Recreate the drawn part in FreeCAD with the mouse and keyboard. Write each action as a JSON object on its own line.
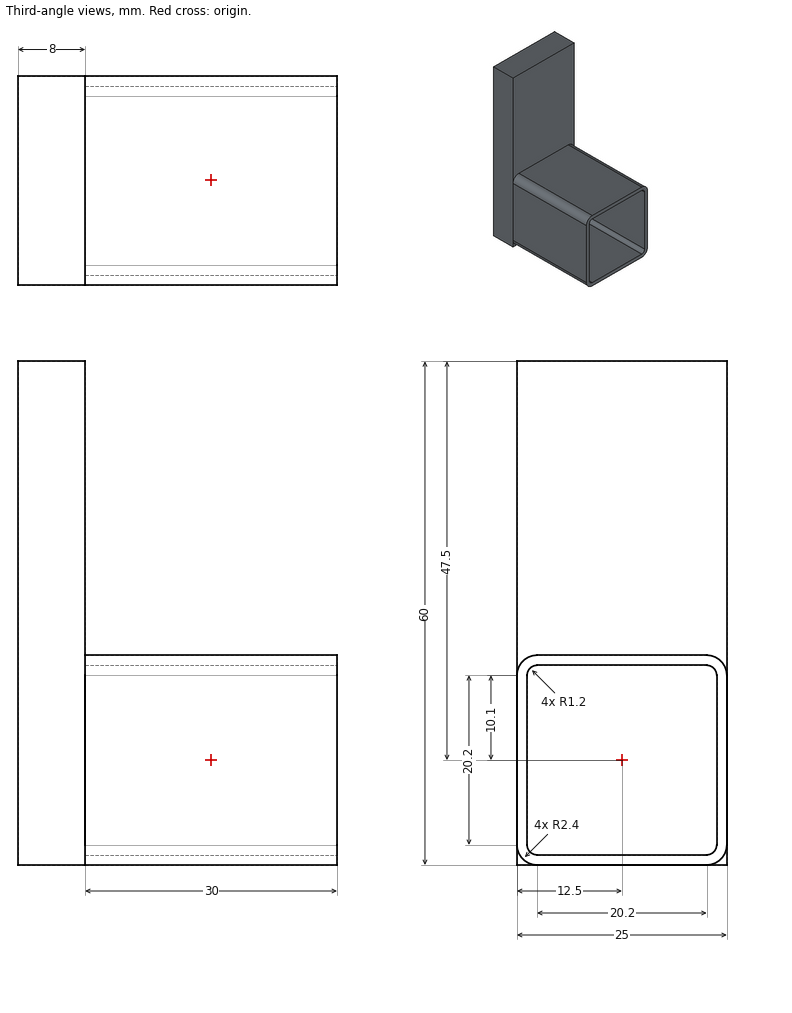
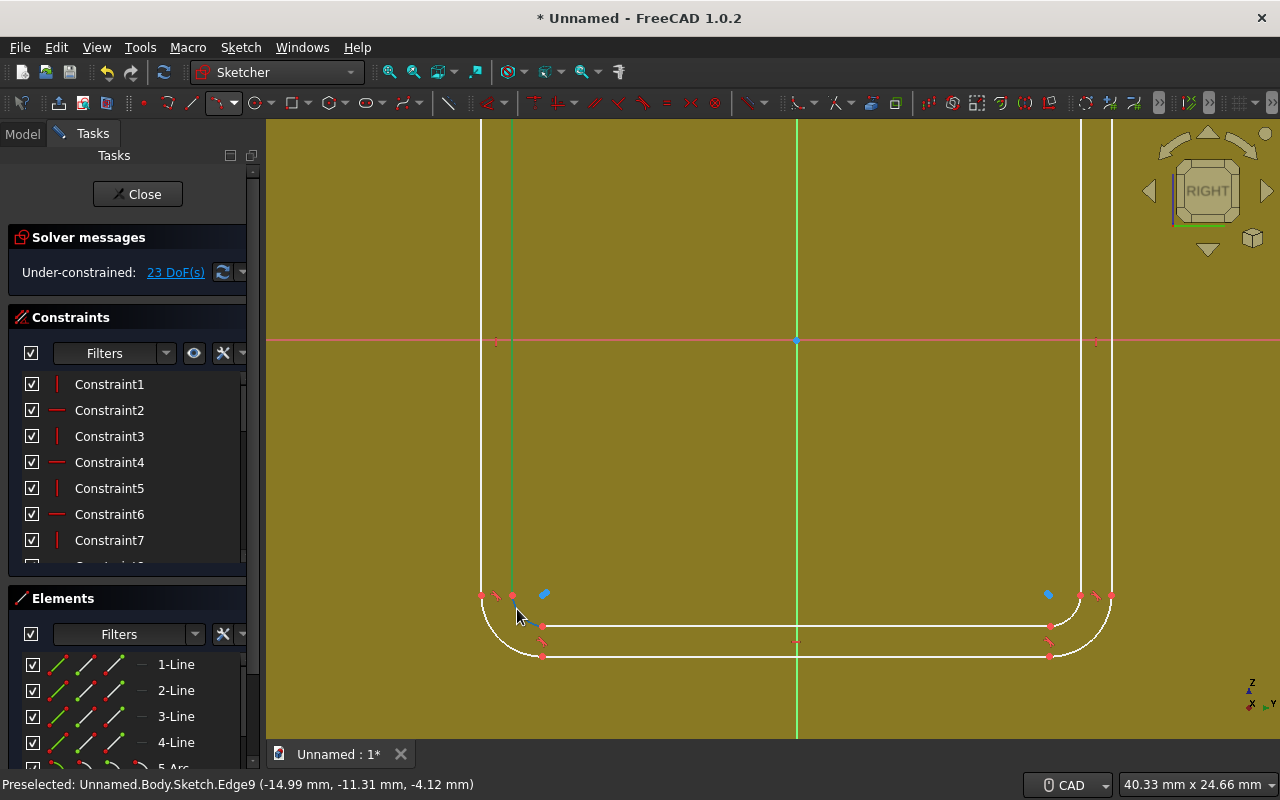
{"action": "left_click", "coordinate": [516, 609]}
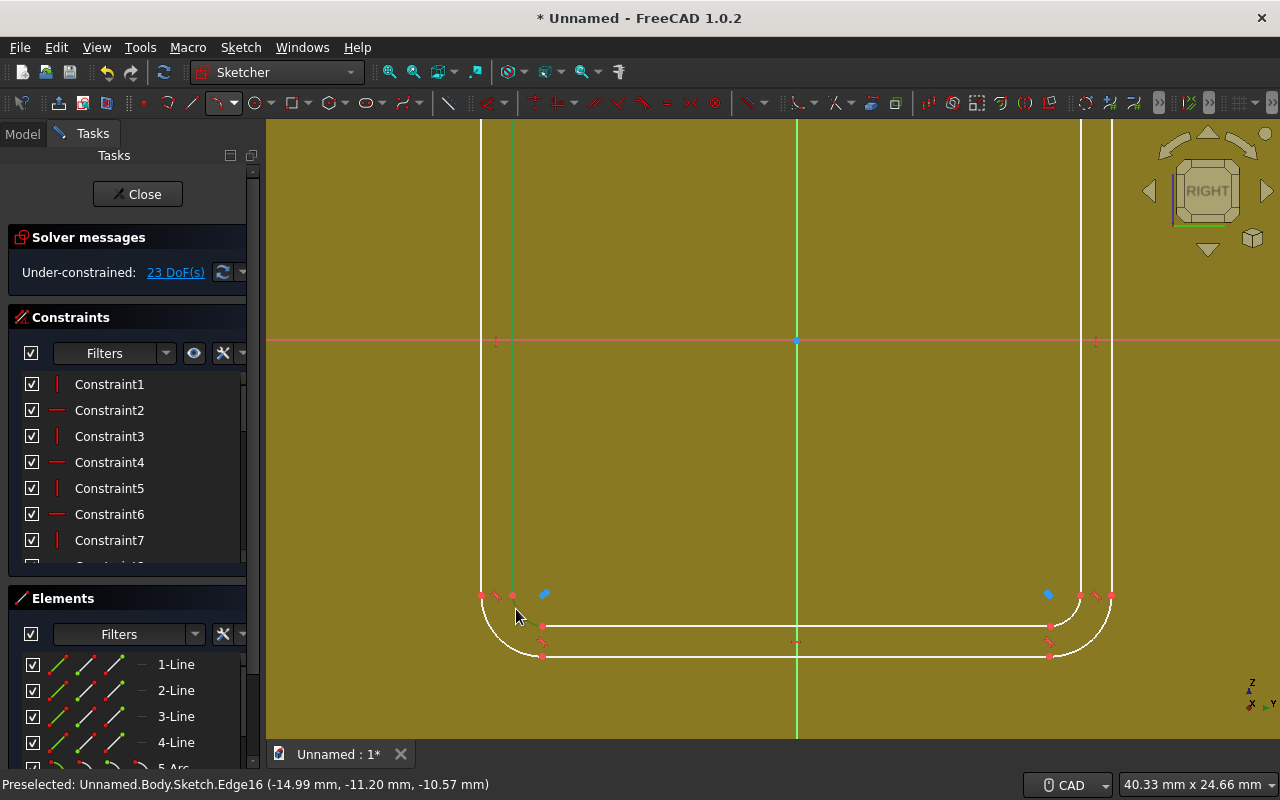
{"action": "key", "text": "t"}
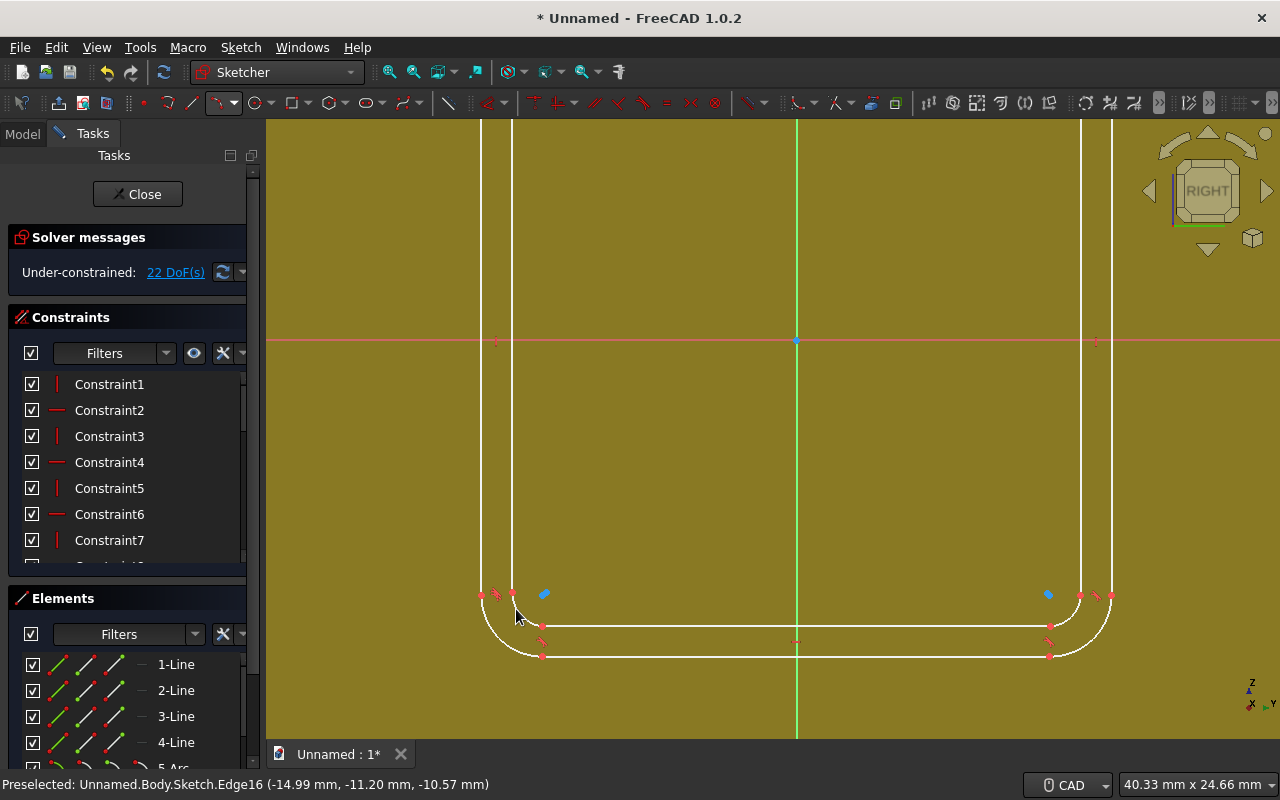
{"action": "scroll", "coordinate": [517, 609], "scroll_direction": "down", "scroll_amount": 2}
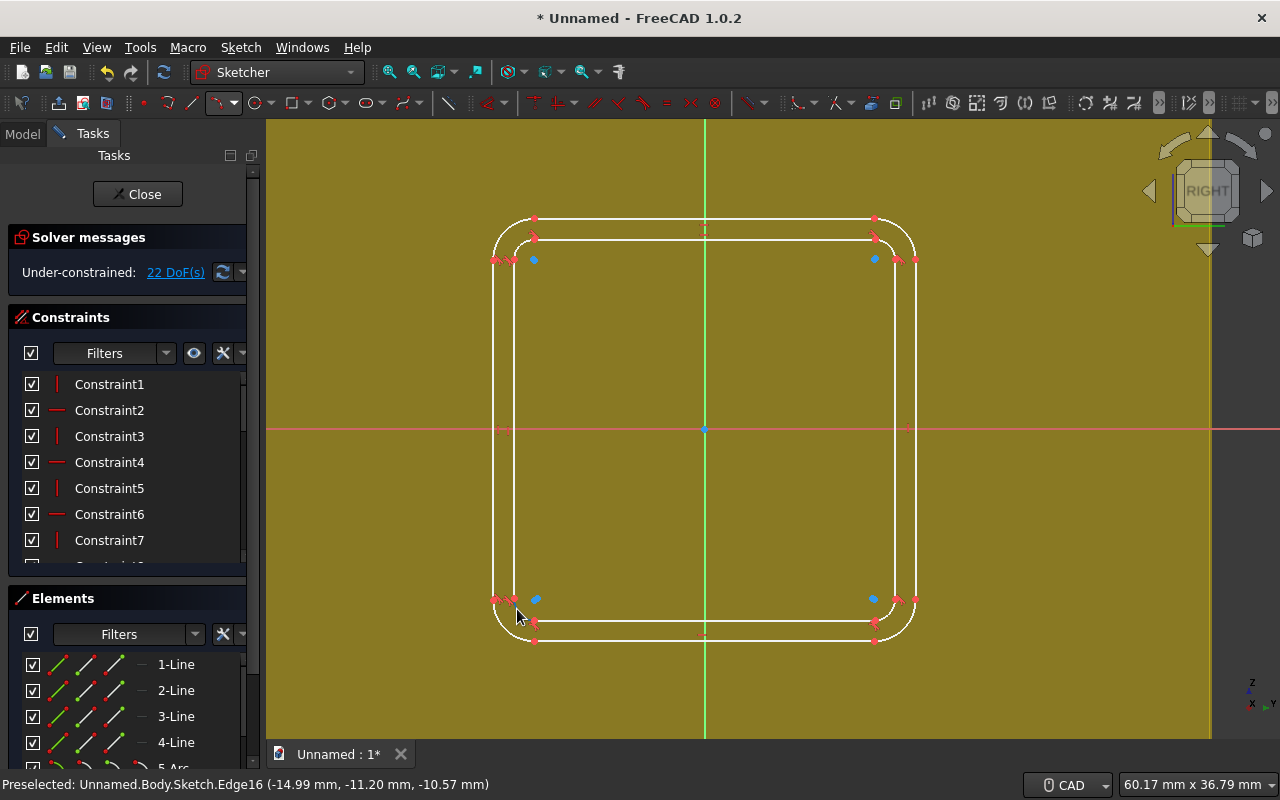
{"action": "left_click", "coordinate": [636, 240]}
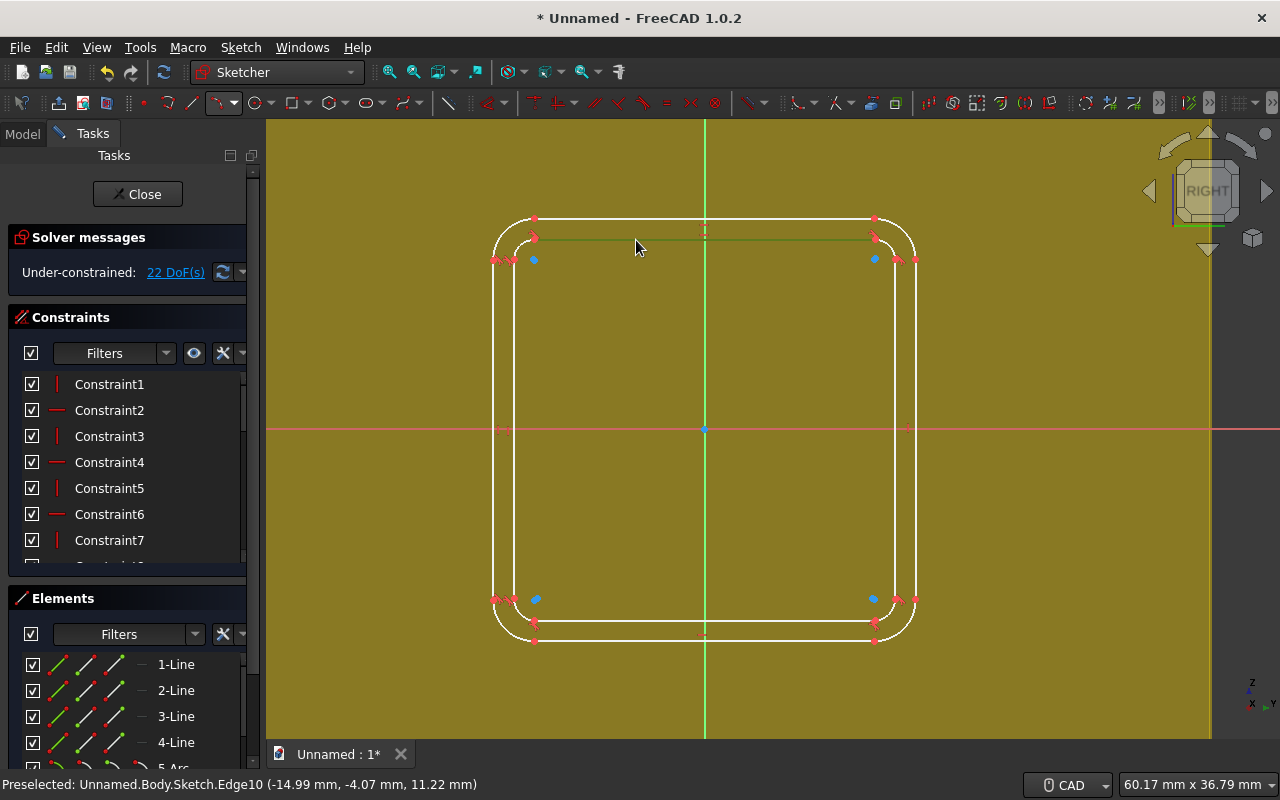
{"action": "scroll", "coordinate": [525, 242], "scroll_direction": "up", "scroll_amount": 2}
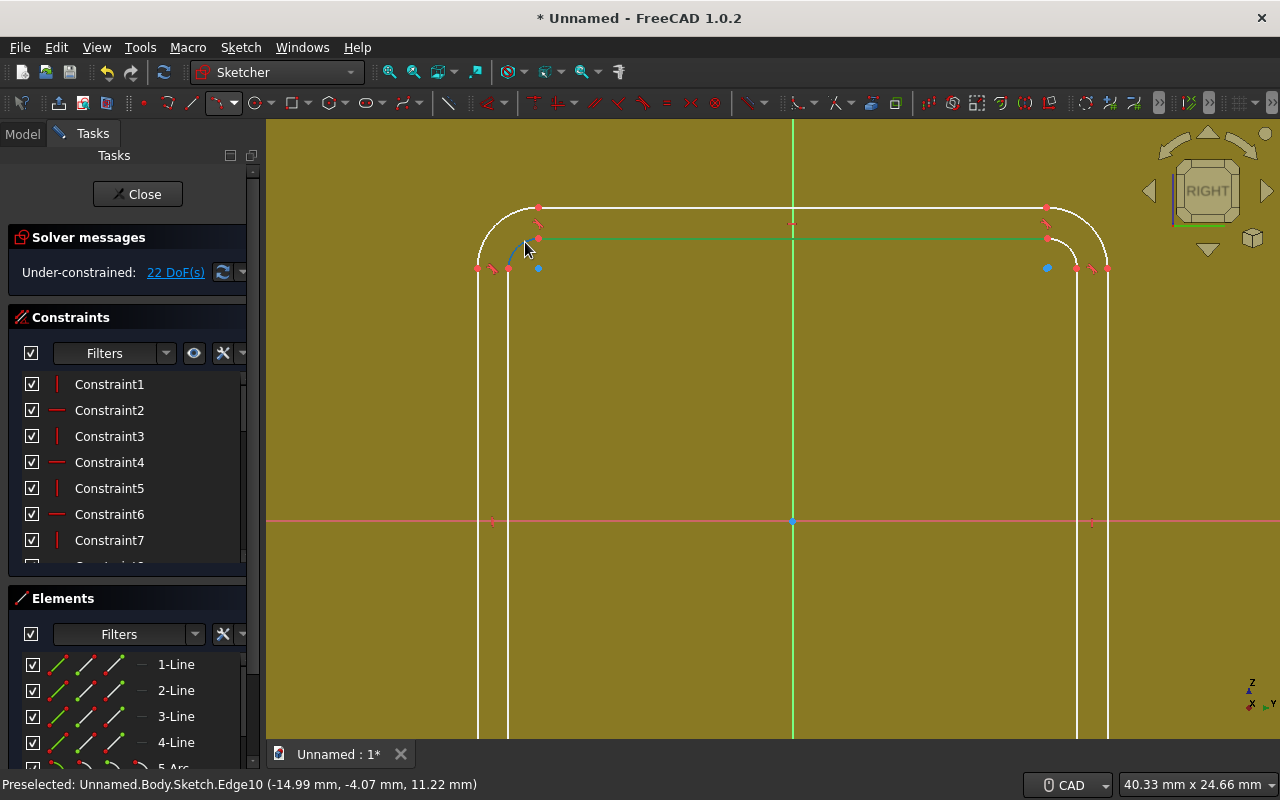
{"action": "left_click", "coordinate": [525, 242]}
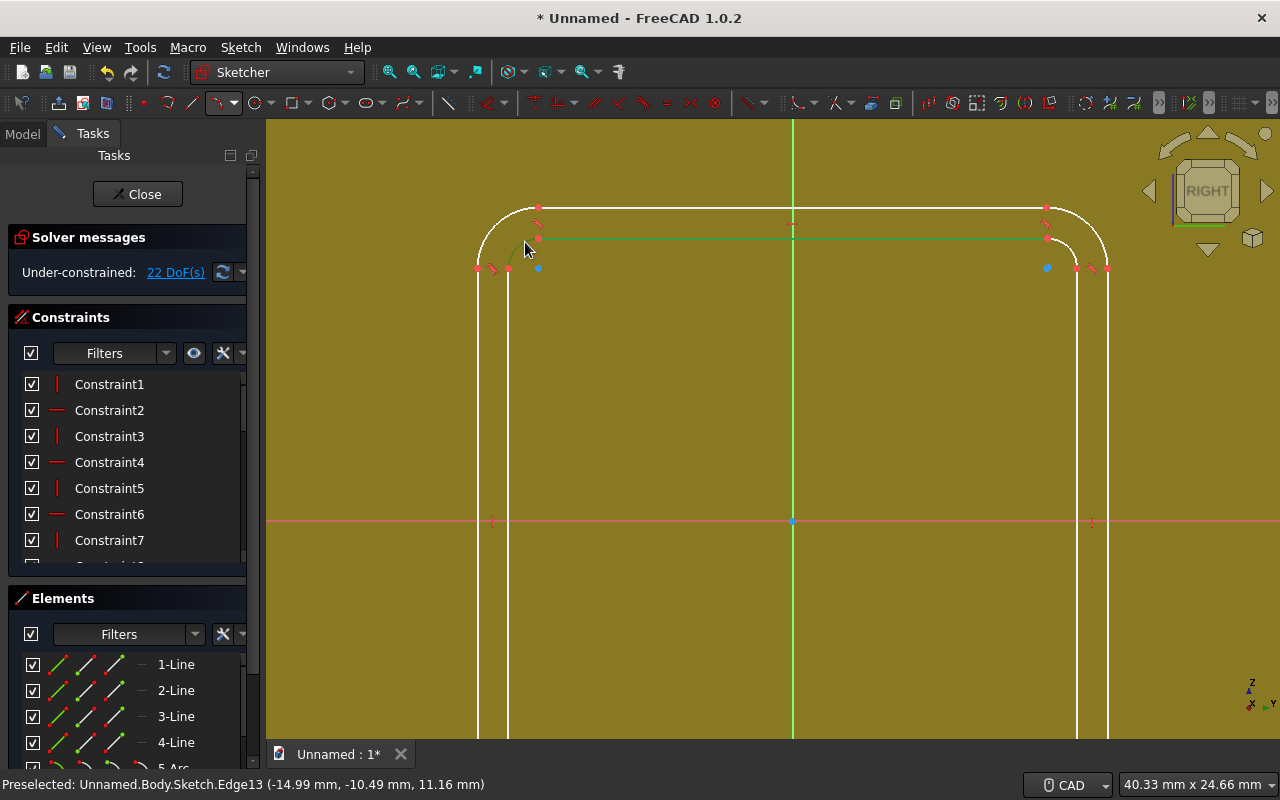
{"action": "left_click", "coordinate": [644, 104]}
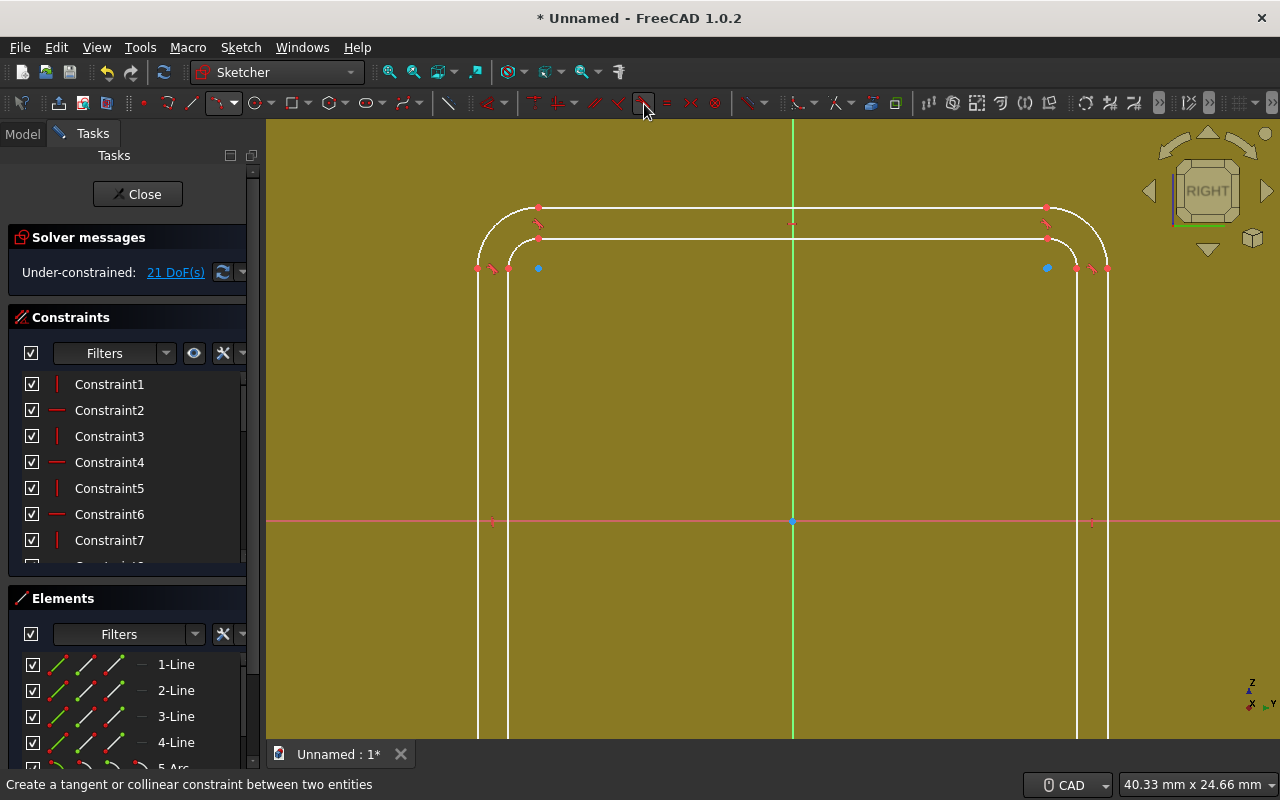
{"action": "left_click", "coordinate": [691, 239]}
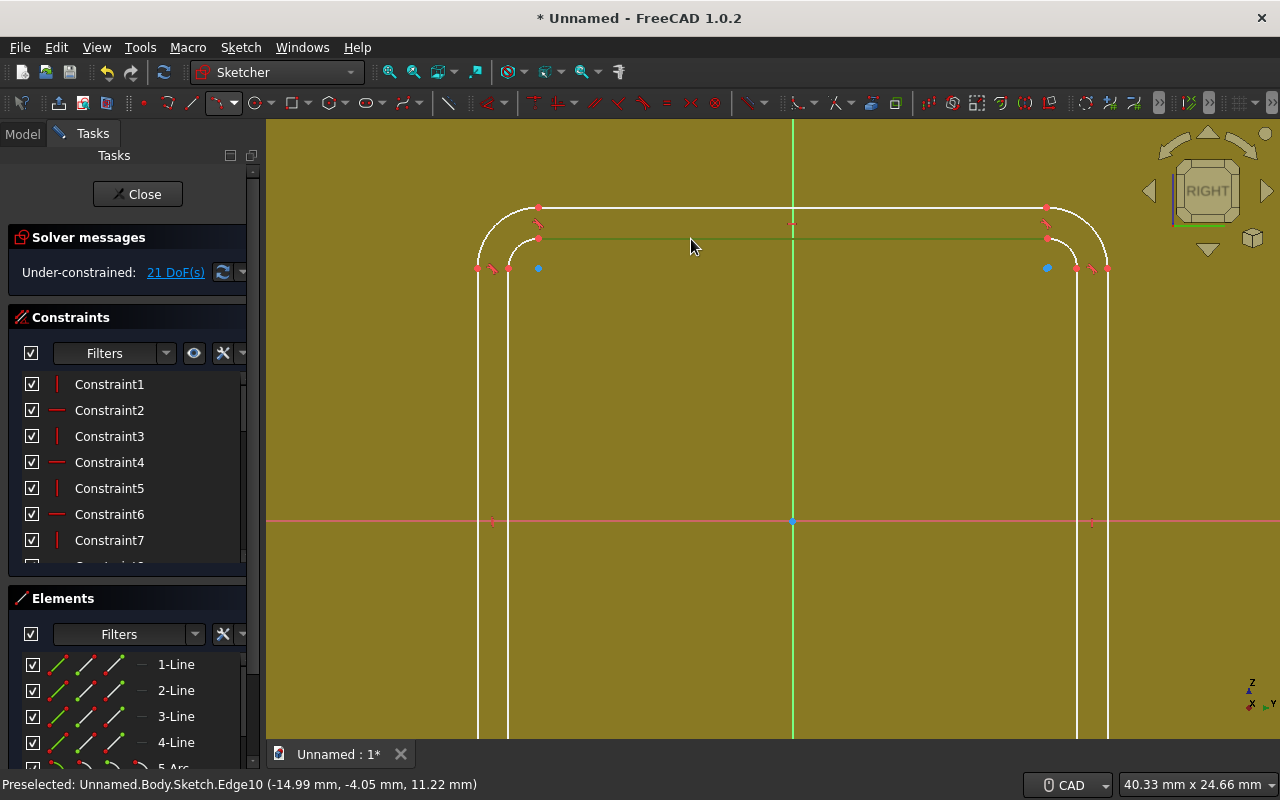
{"action": "left_click", "coordinate": [1074, 255]}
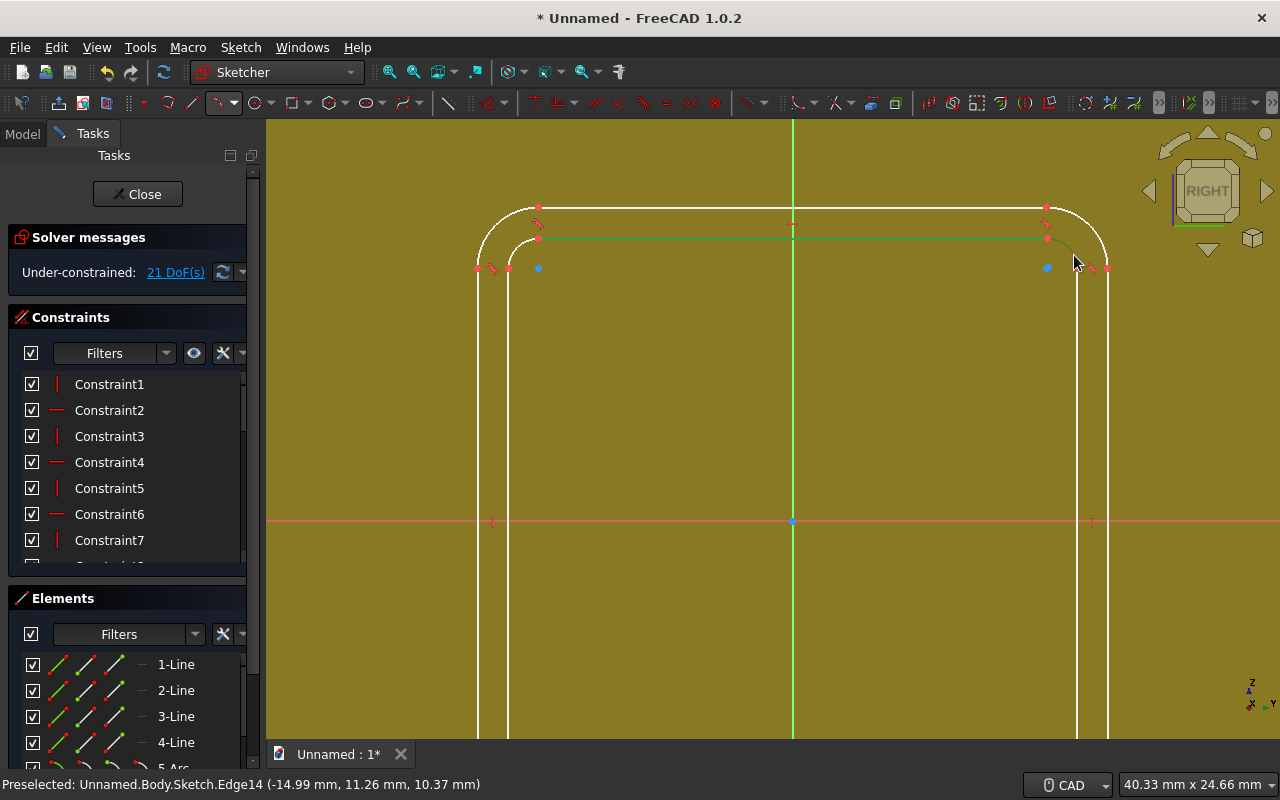
{"action": "key", "text": "t"}